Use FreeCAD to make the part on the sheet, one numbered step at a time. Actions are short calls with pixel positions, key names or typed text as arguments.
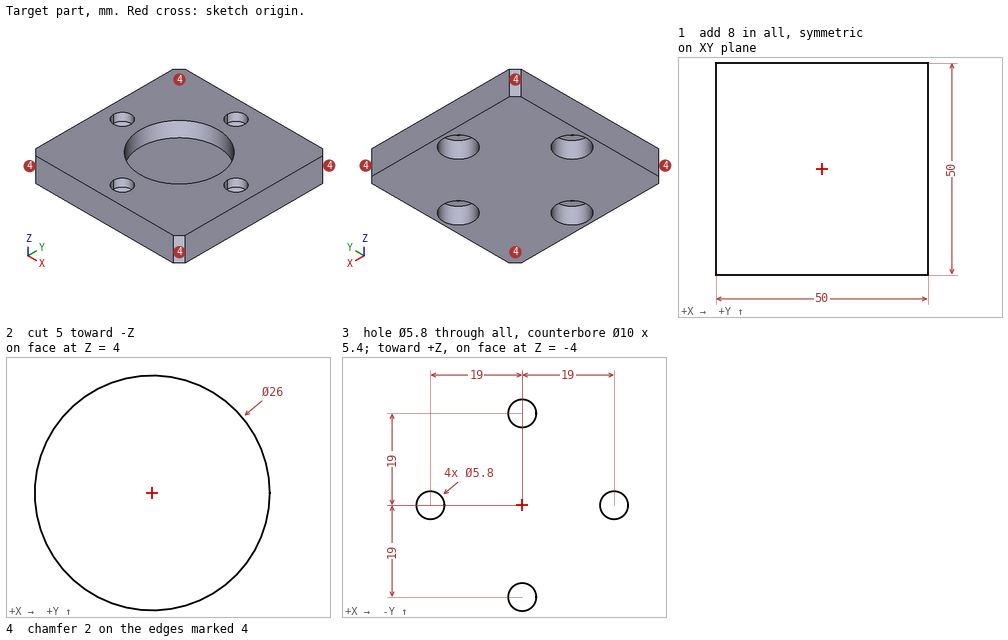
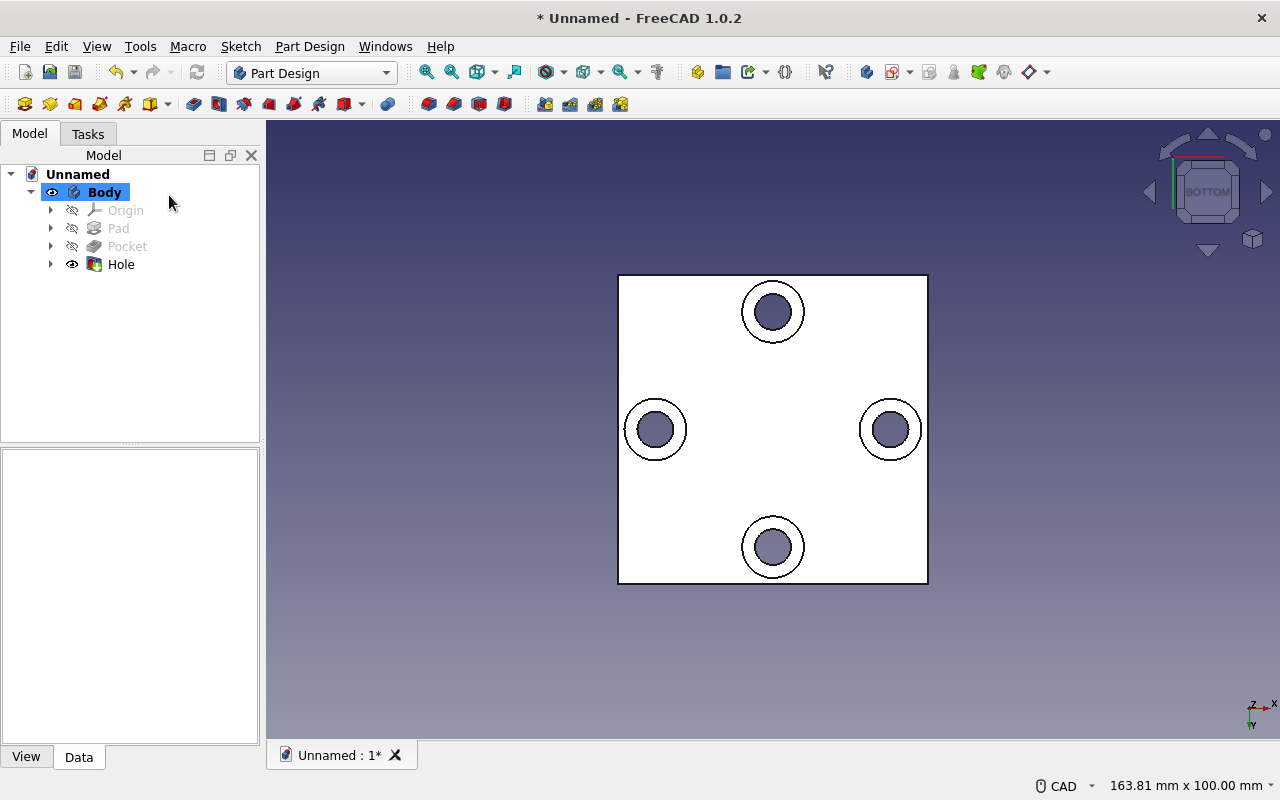
key(0)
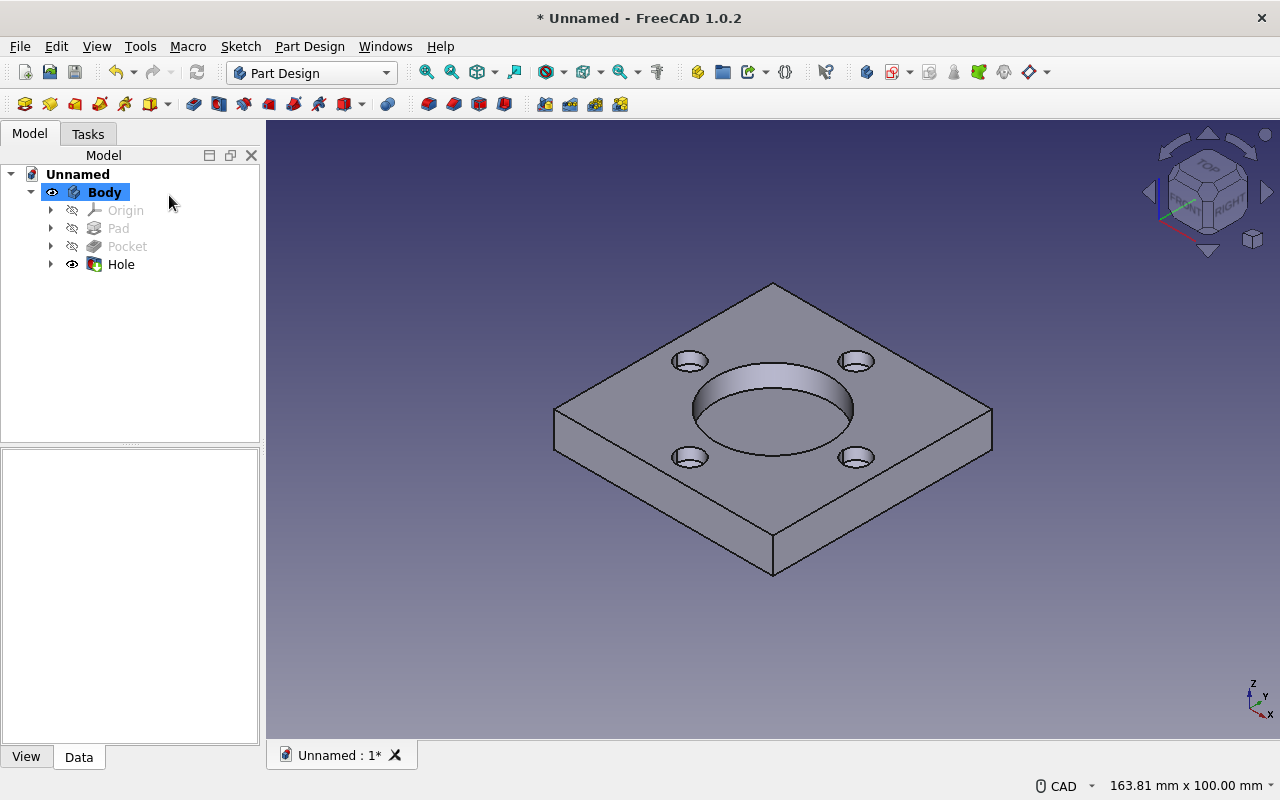
click(773, 555)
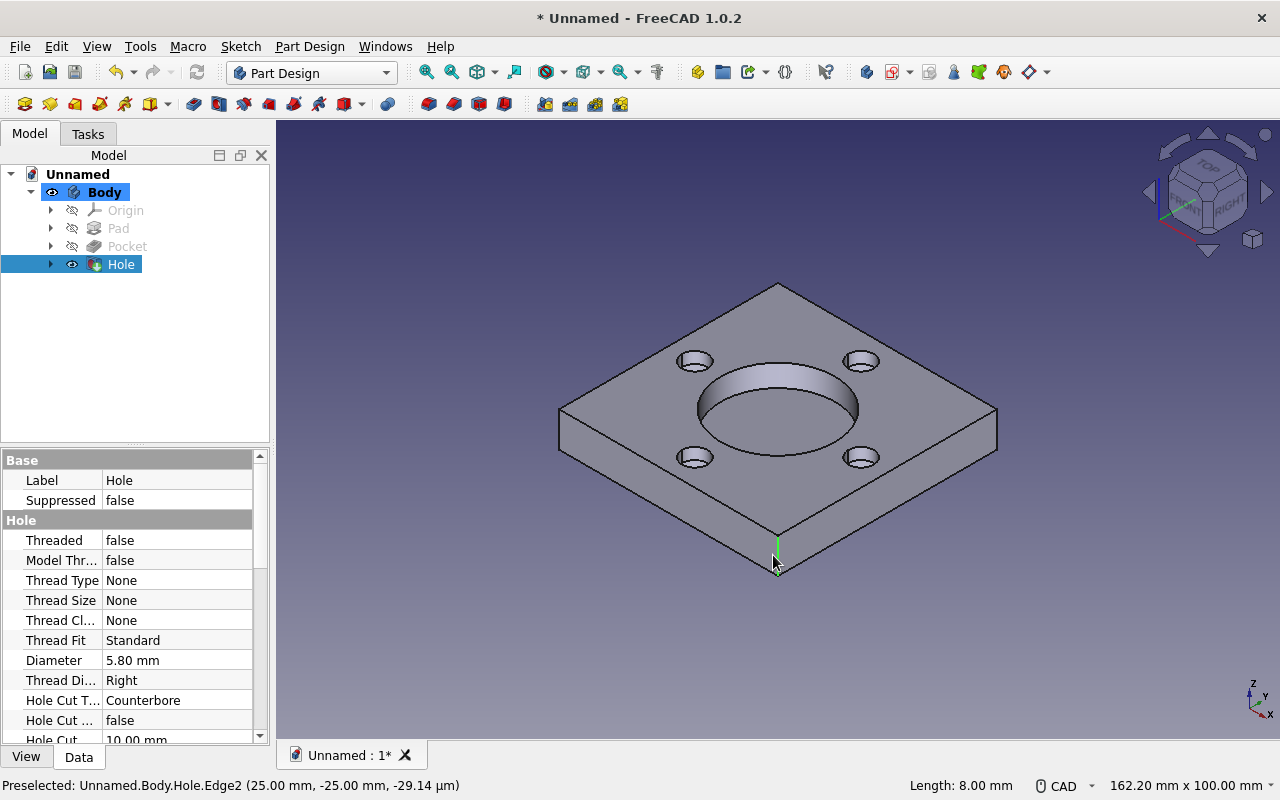
key(2)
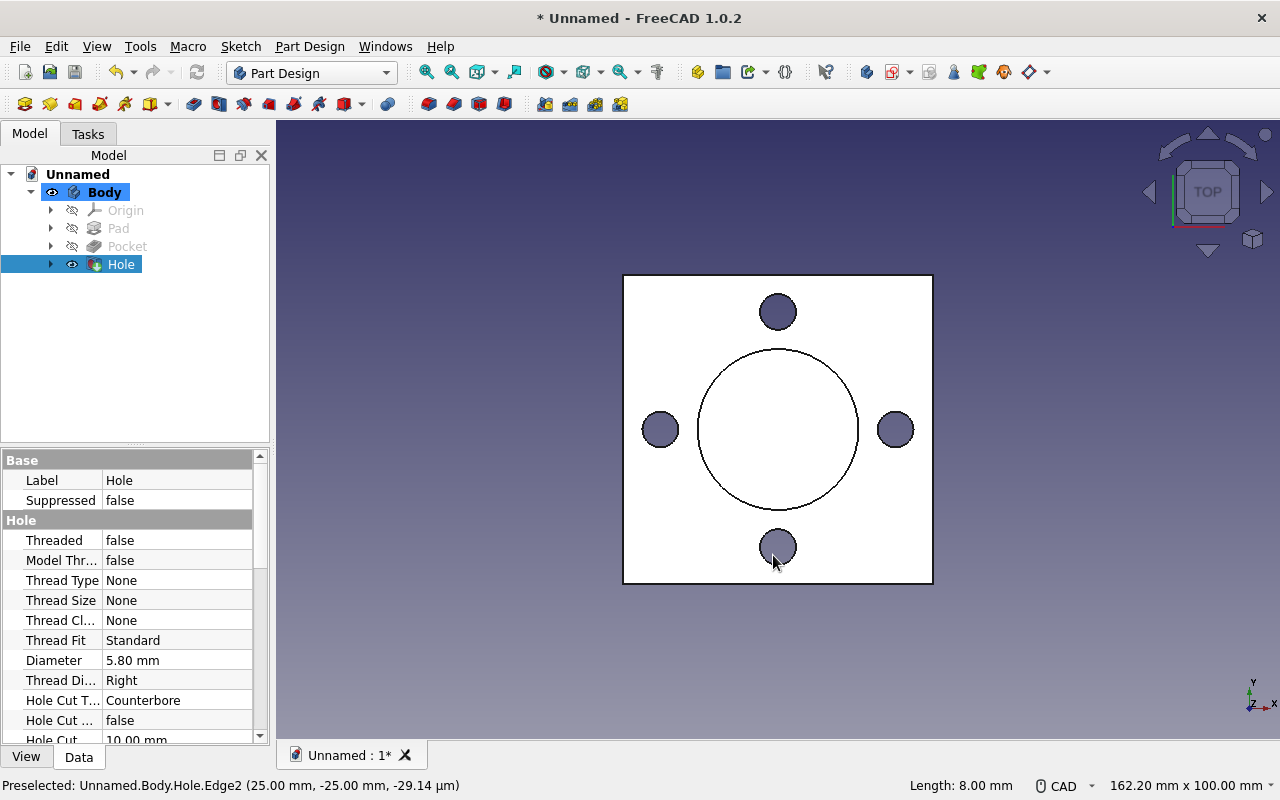
key(1)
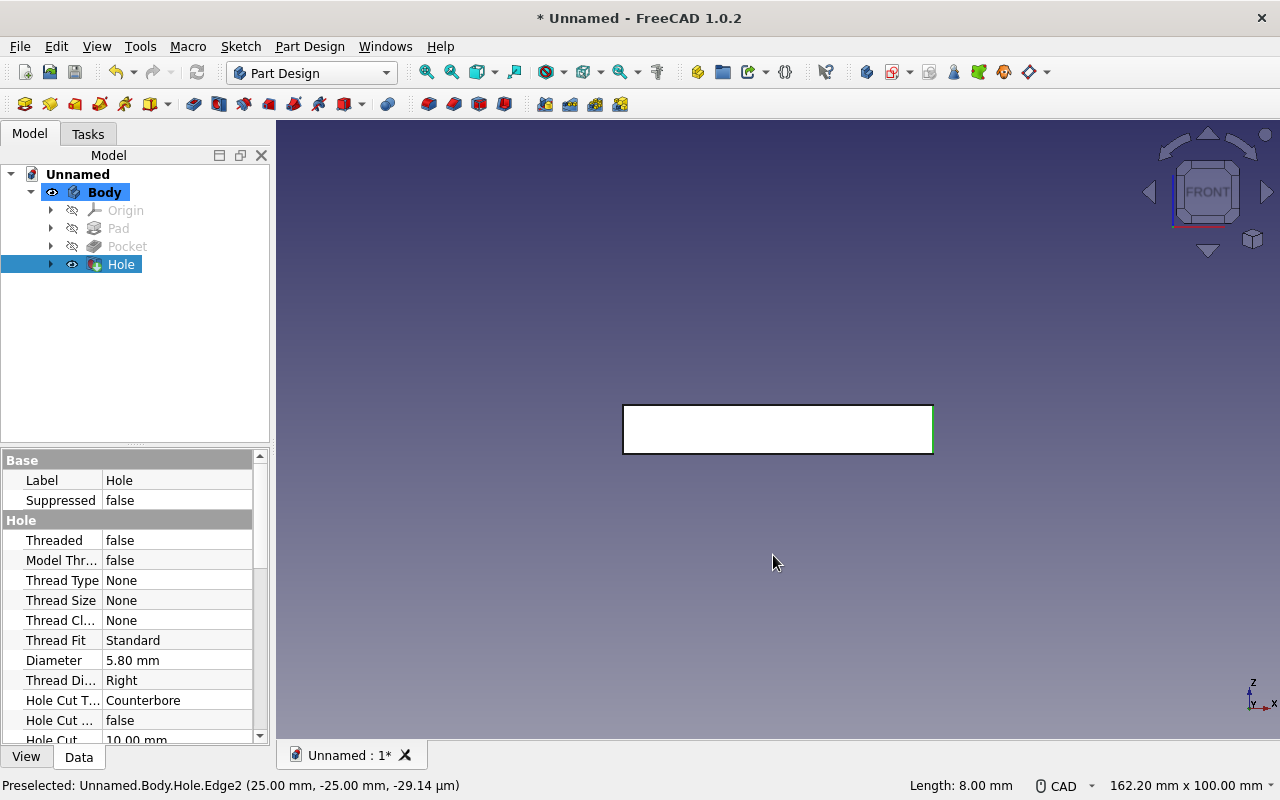
click(427, 72)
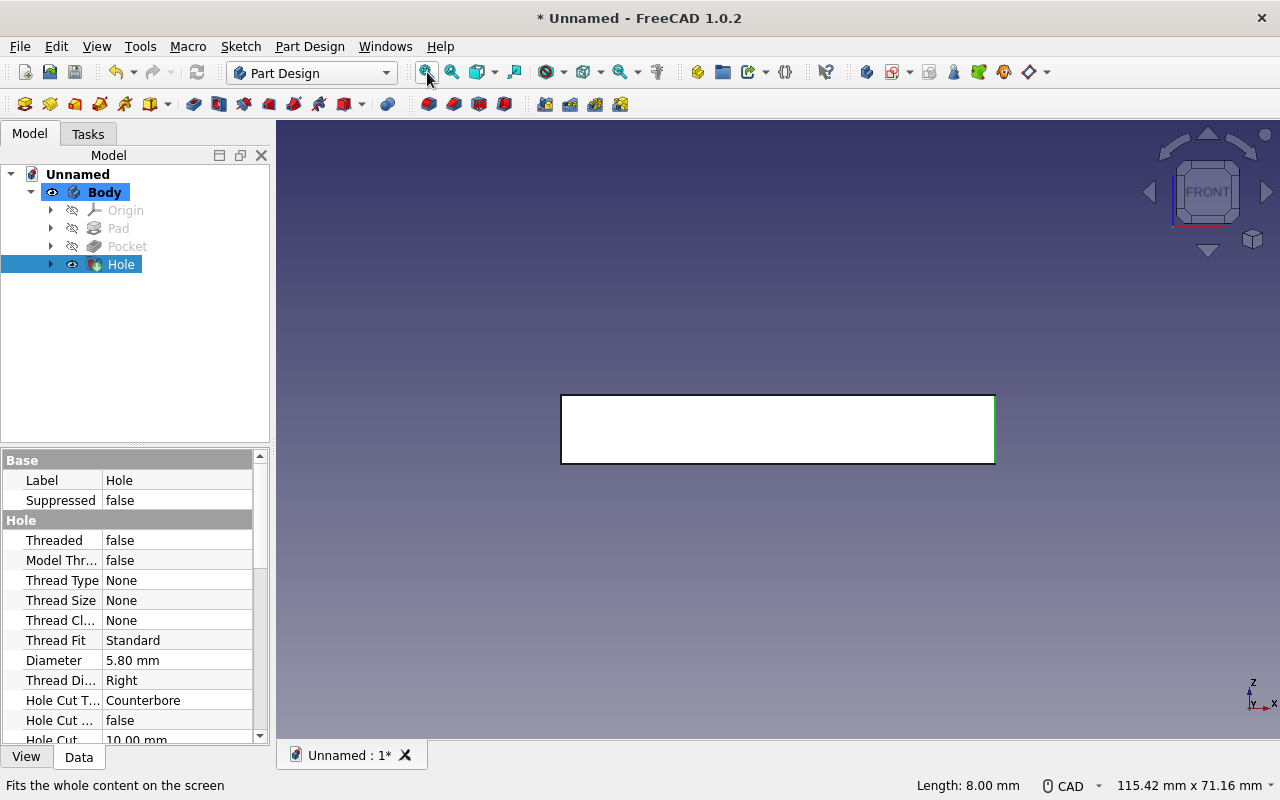
click(561, 429, ctrl)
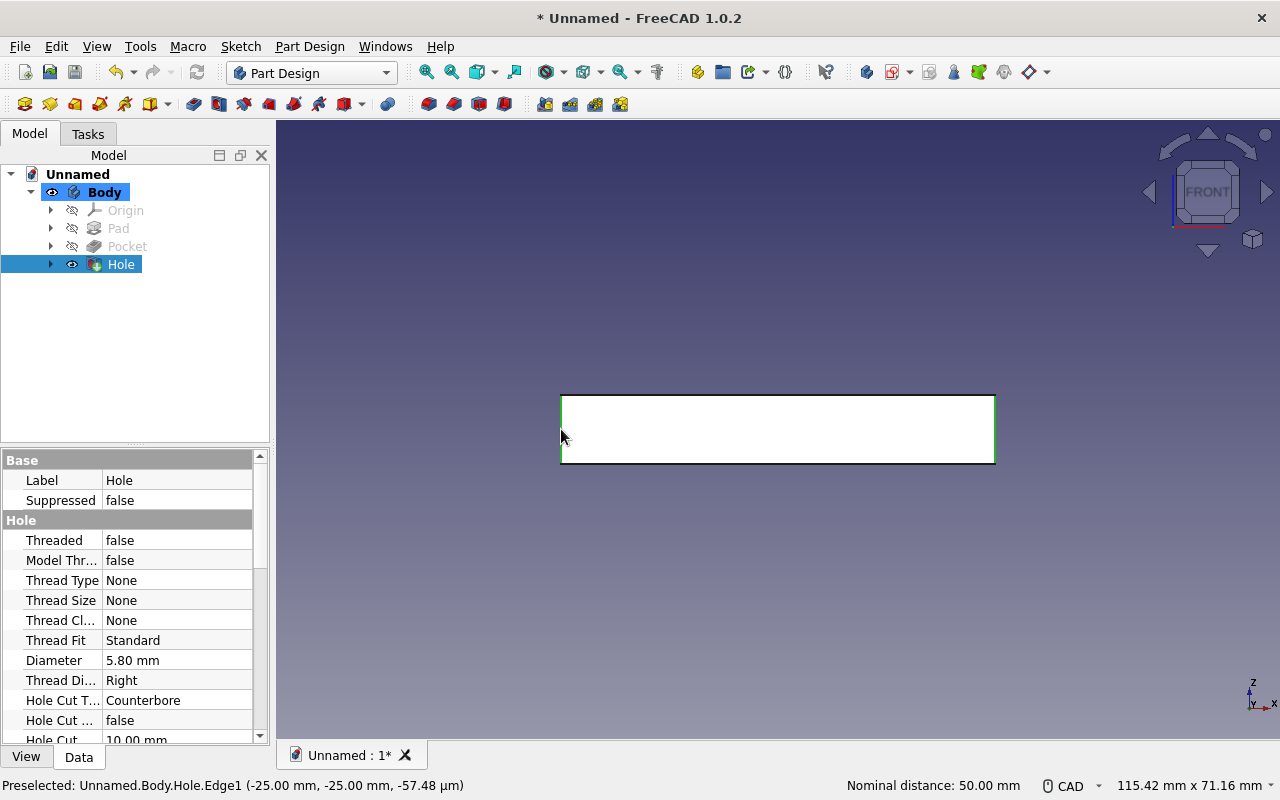
key(3)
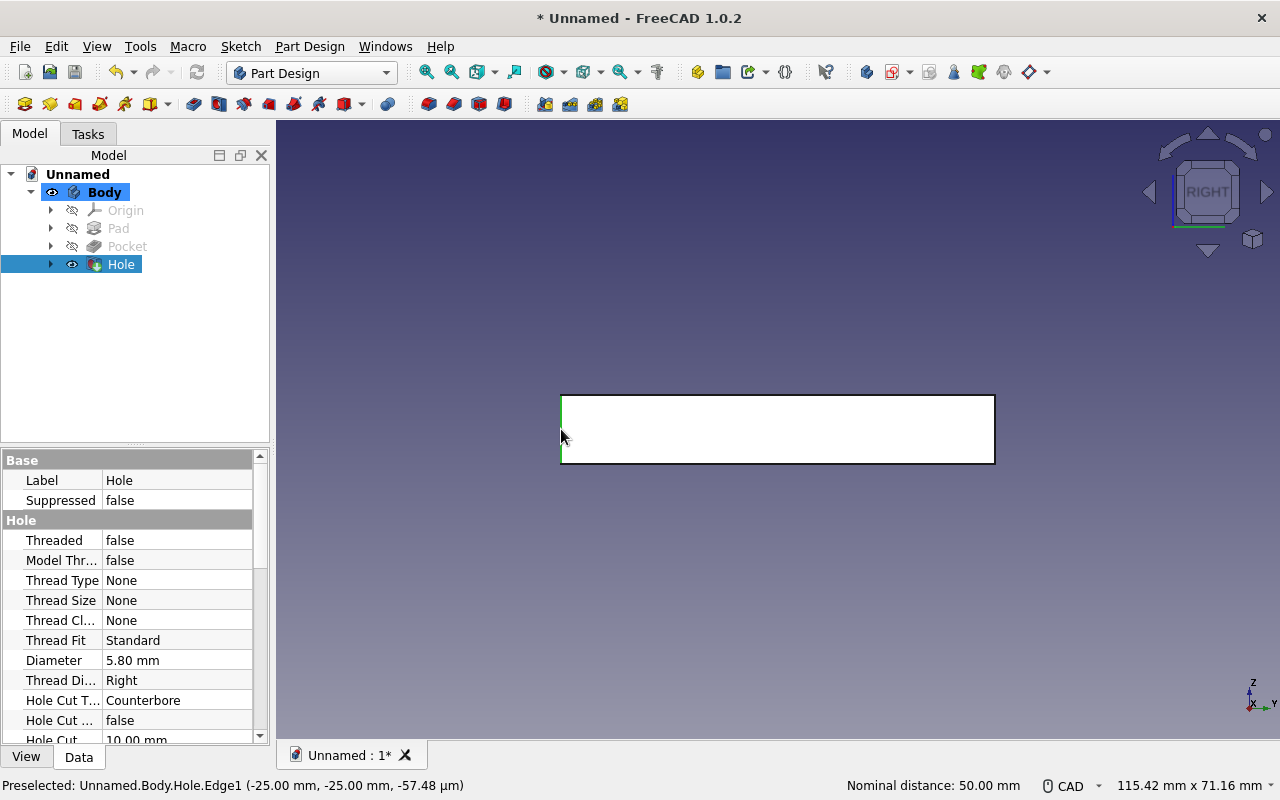
click(427, 72)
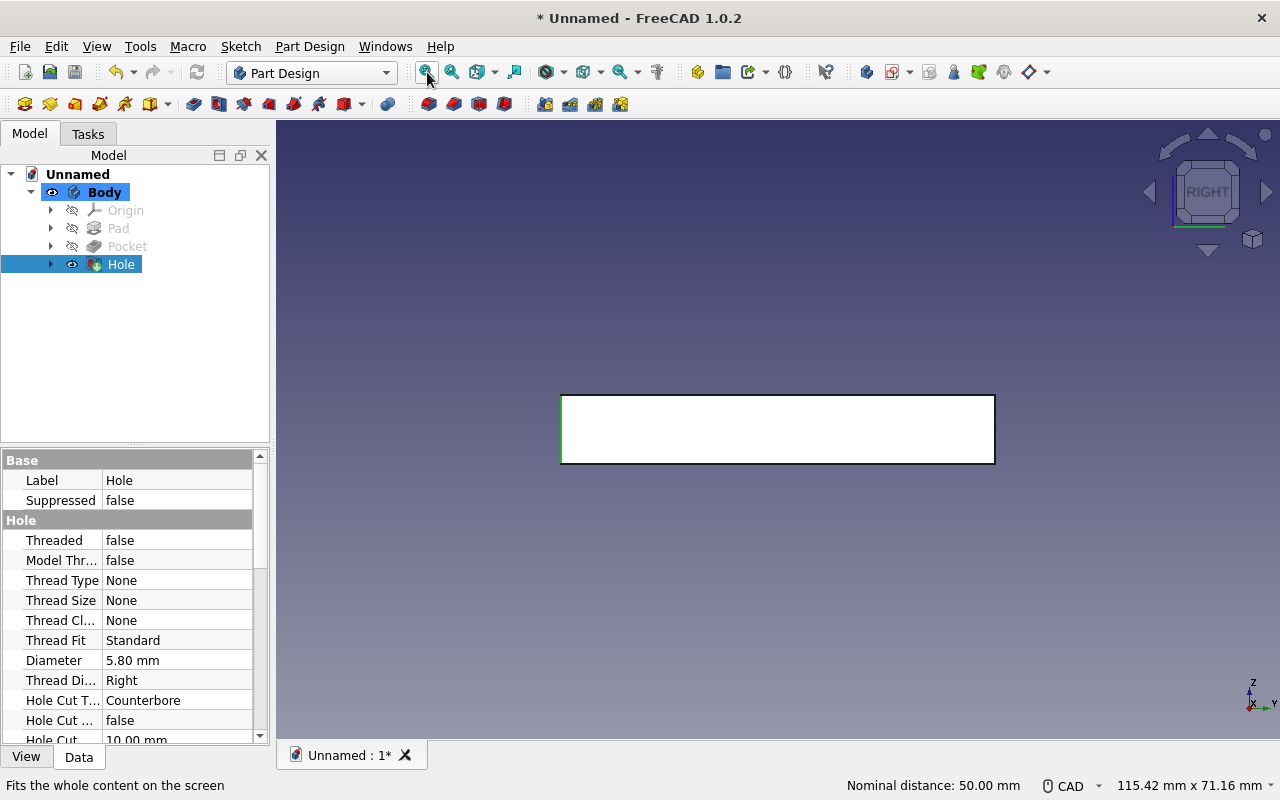
click(995, 428, ctrl)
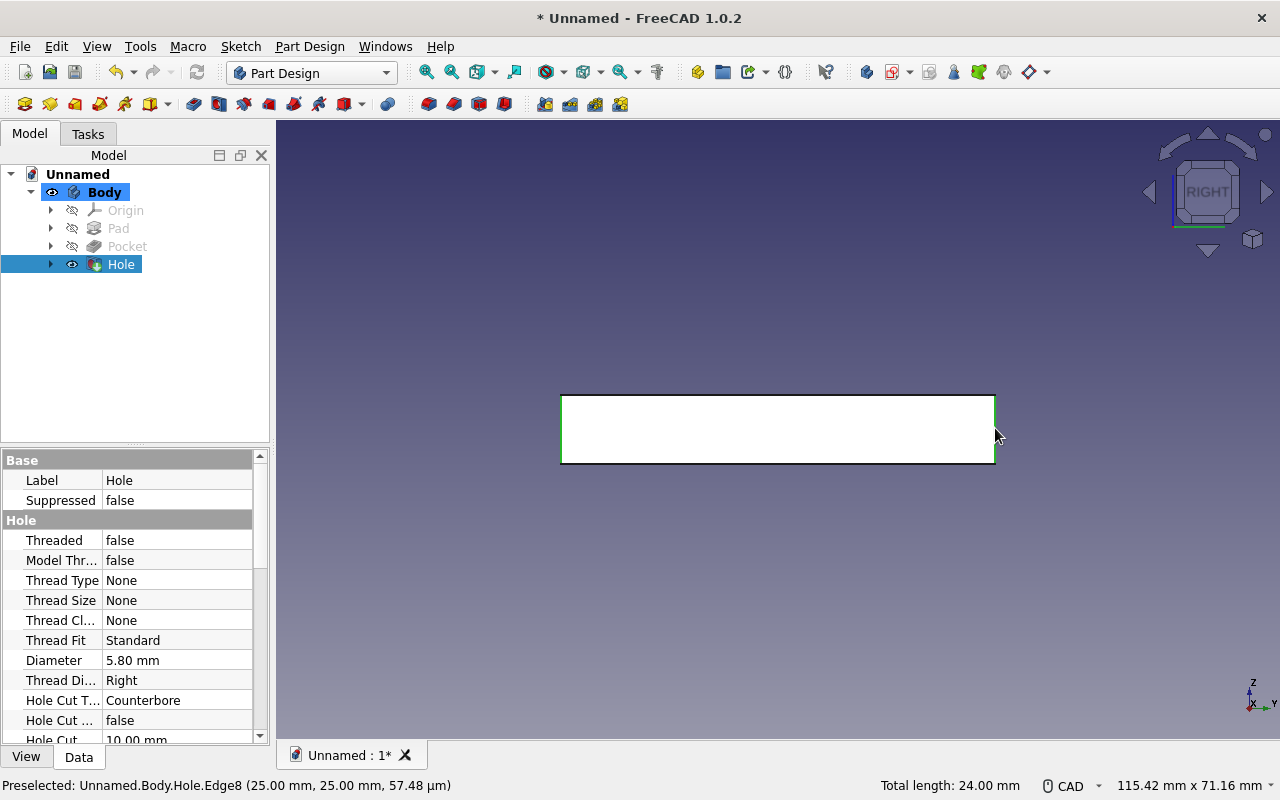
key(5)